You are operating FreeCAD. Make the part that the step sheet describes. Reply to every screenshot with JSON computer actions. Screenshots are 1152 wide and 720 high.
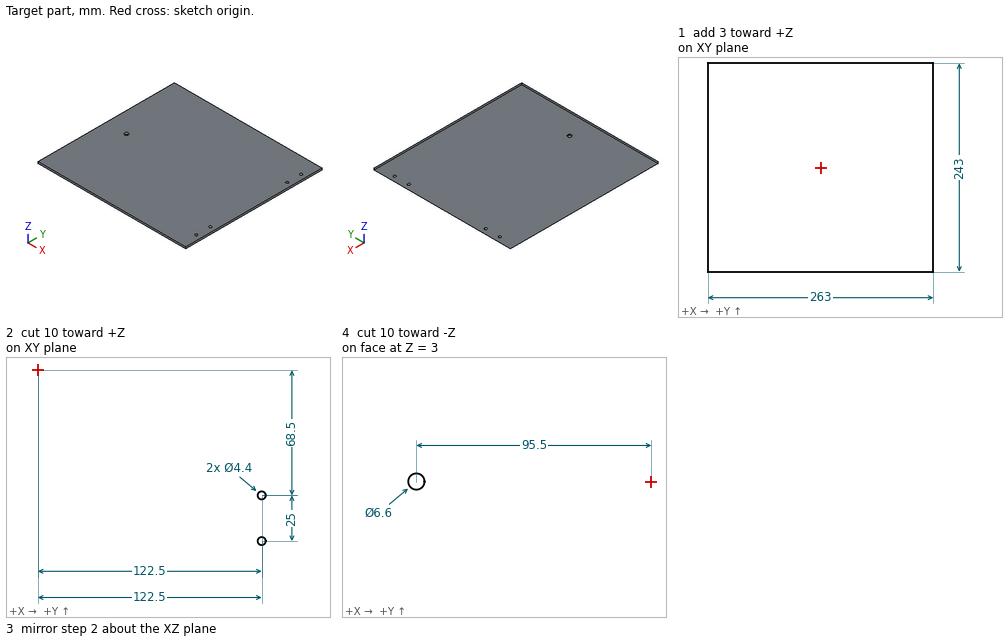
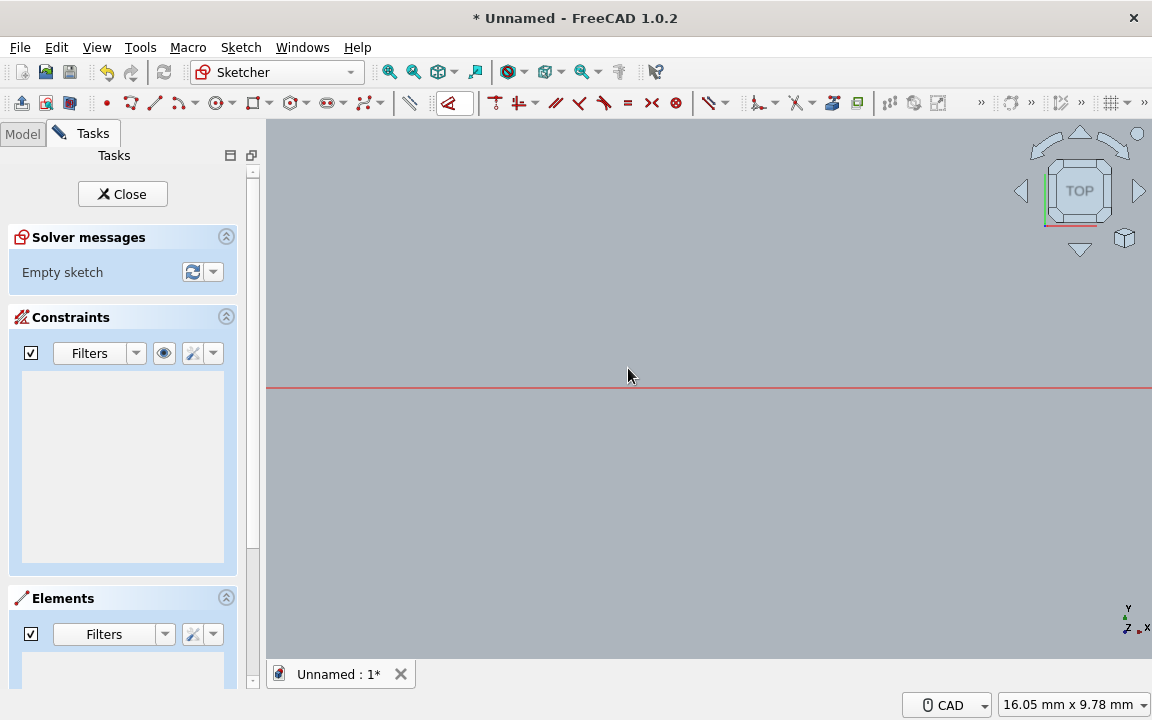
{"action": "key", "text": "g c"}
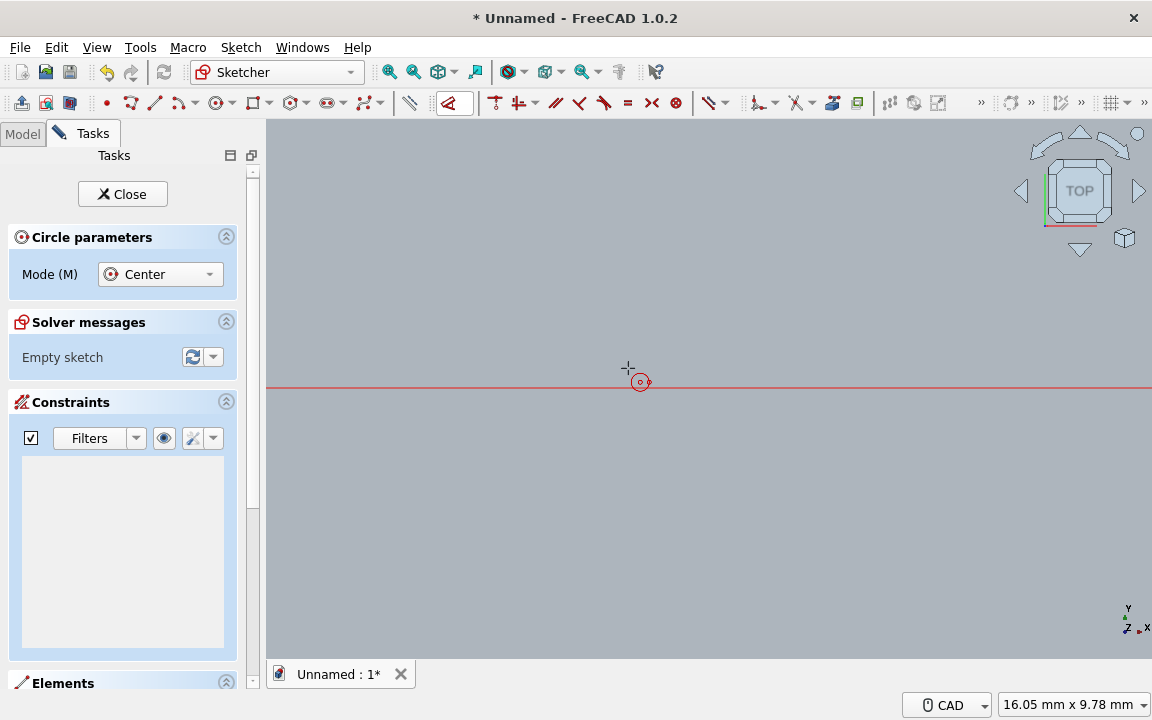
{"action": "left_click", "coordinate": [640, 388]}
{"action": "left_click", "coordinate": [769, 260]}
{"action": "key", "text": "Escape"}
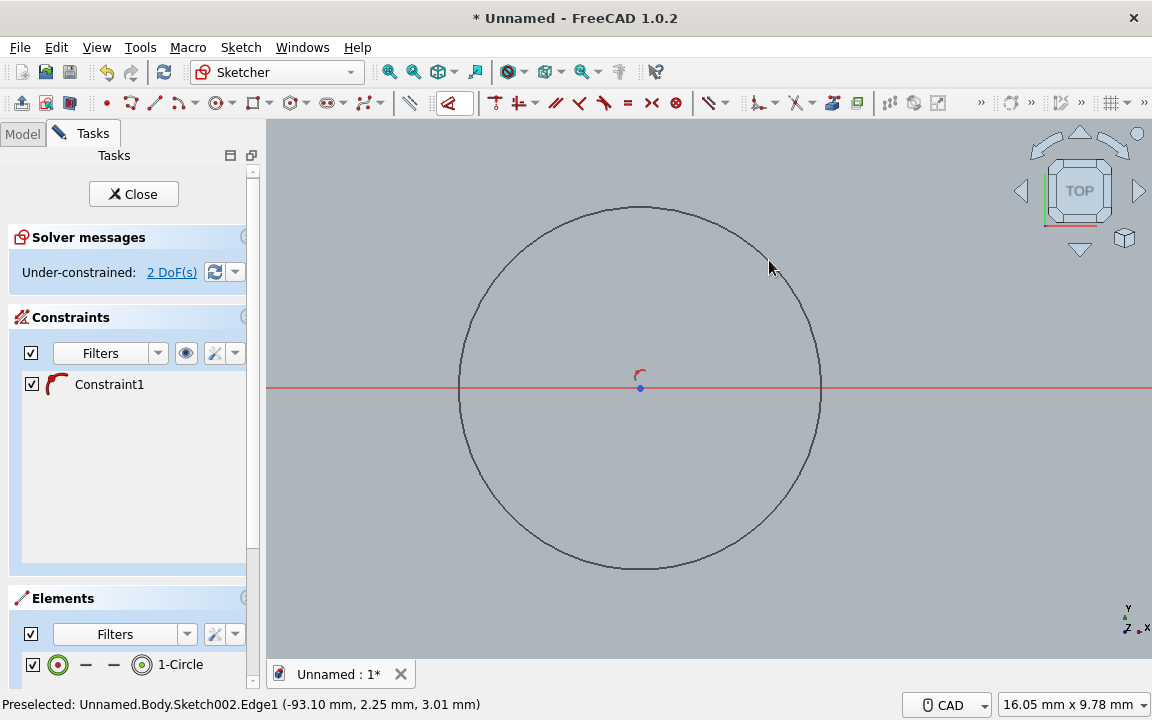
{"action": "left_click", "coordinate": [768, 260]}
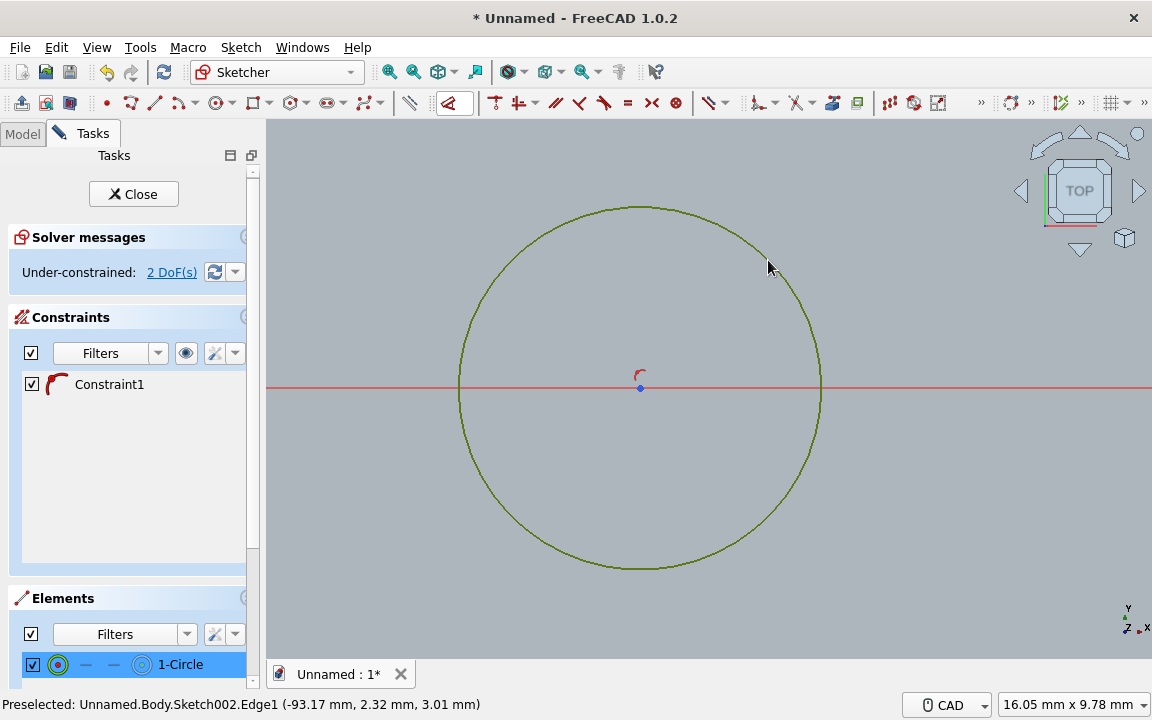
{"action": "key", "text": "k o"}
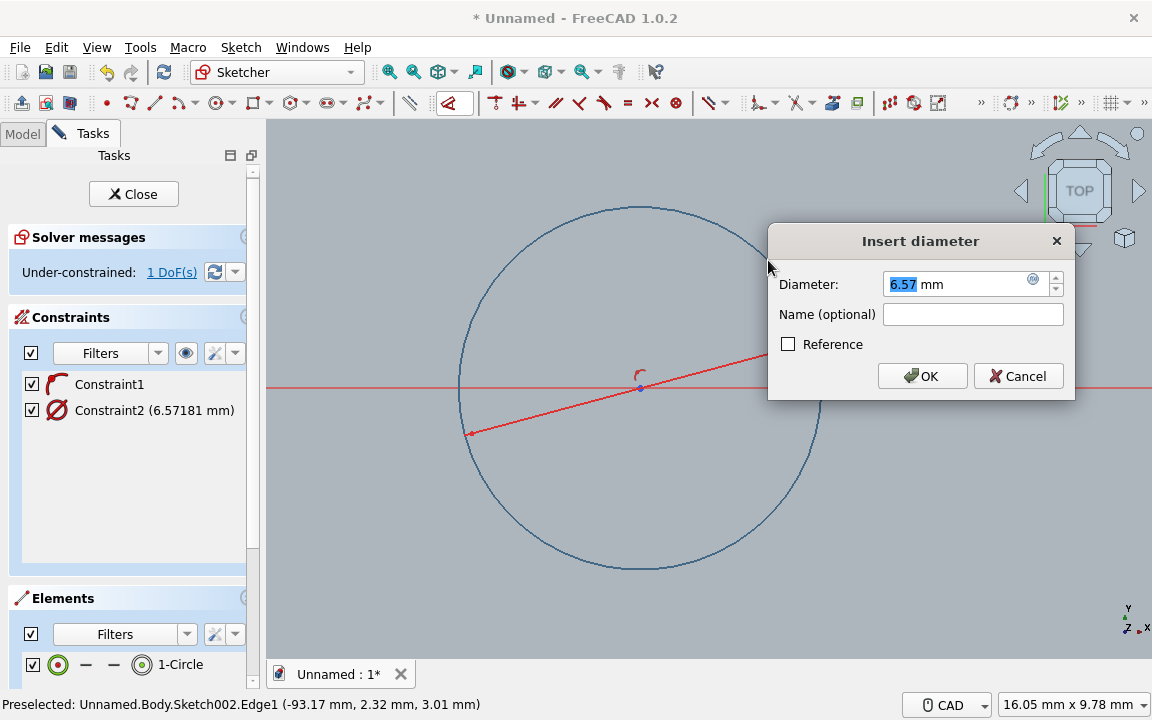
{"action": "type", "text": "6.6"}
{"action": "key", "text": "Return"}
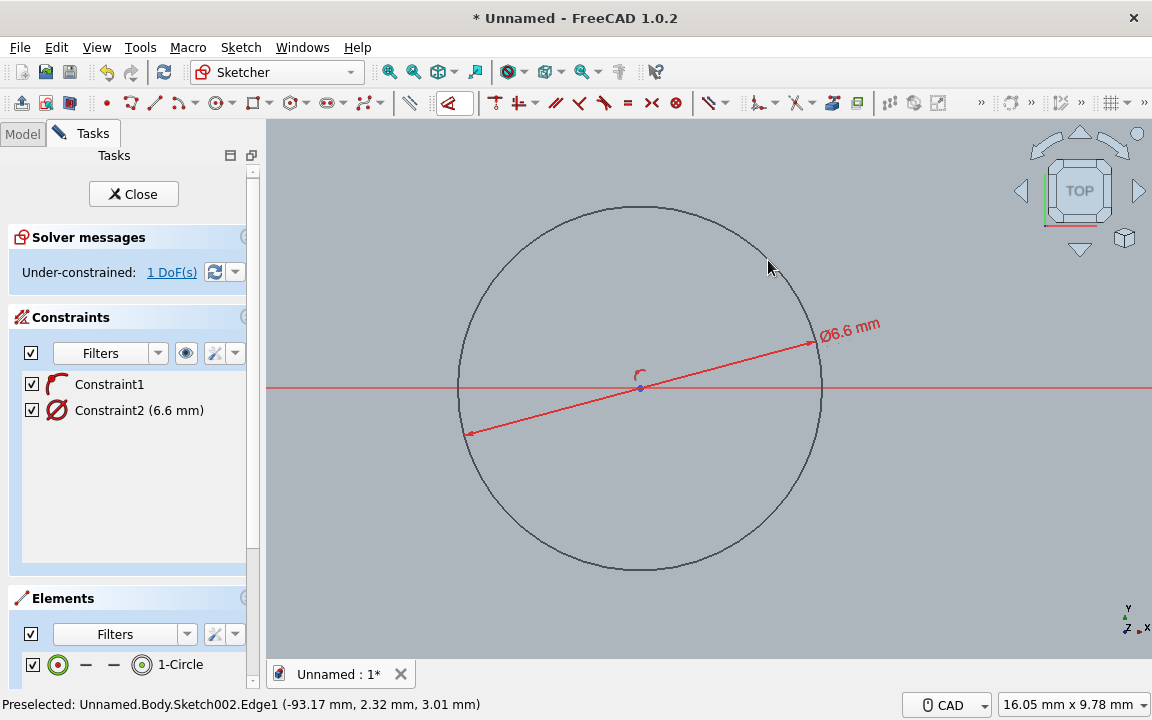
{"action": "left_click", "coordinate": [640, 388]}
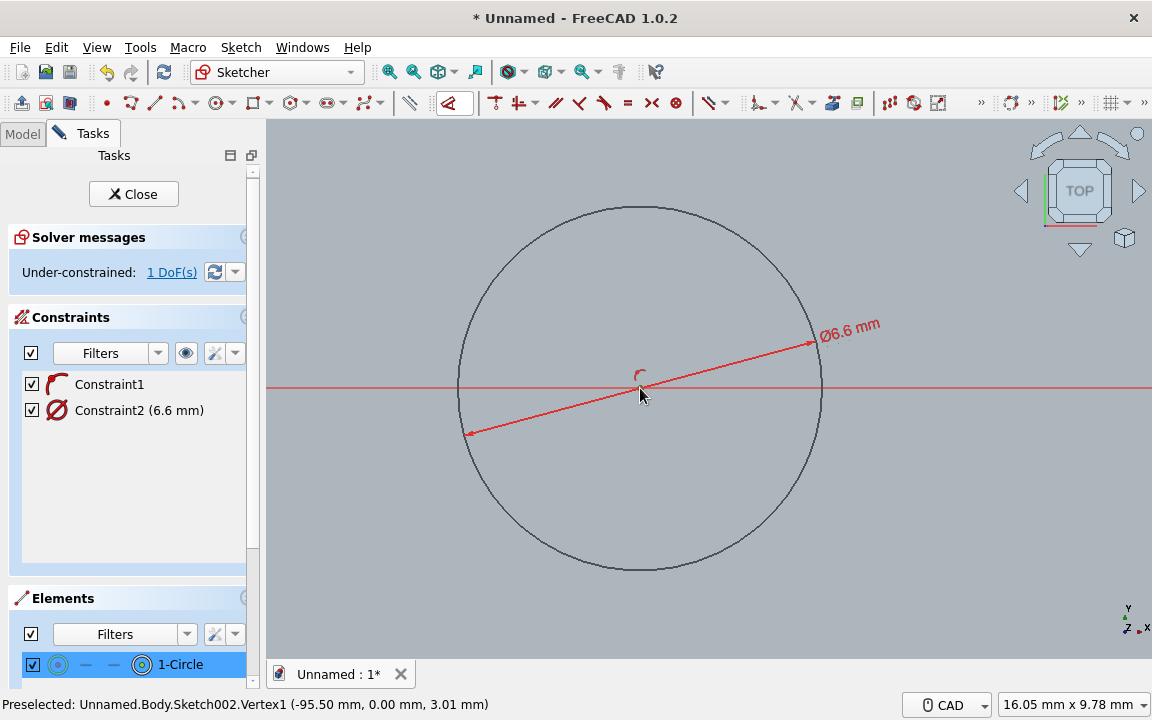
{"action": "key", "text": "l"}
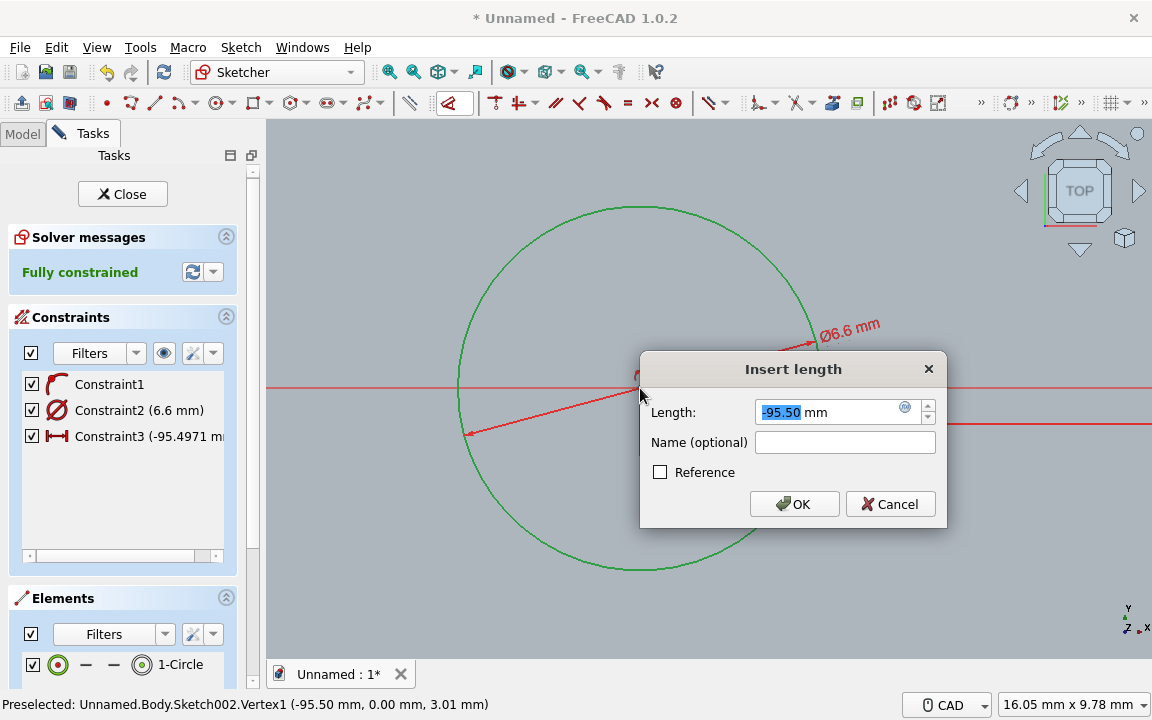
{"action": "type", "text": "-95.5"}
{"action": "key", "text": "Return"}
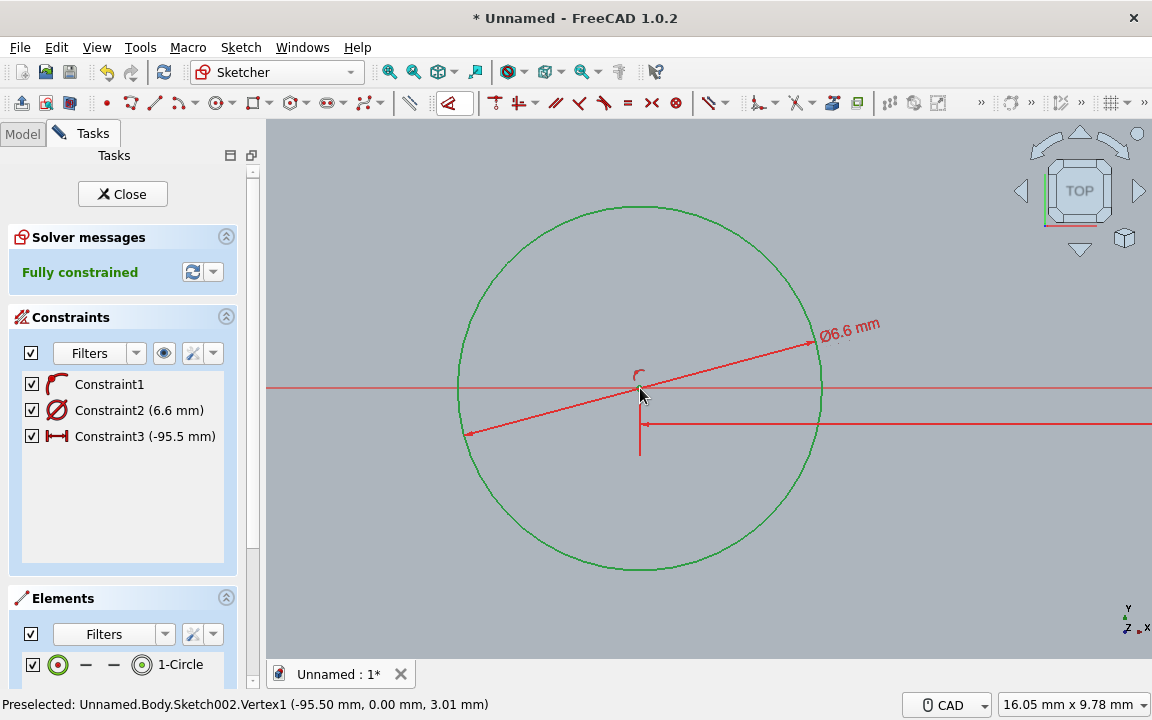
{"action": "left_click", "coordinate": [123, 194]}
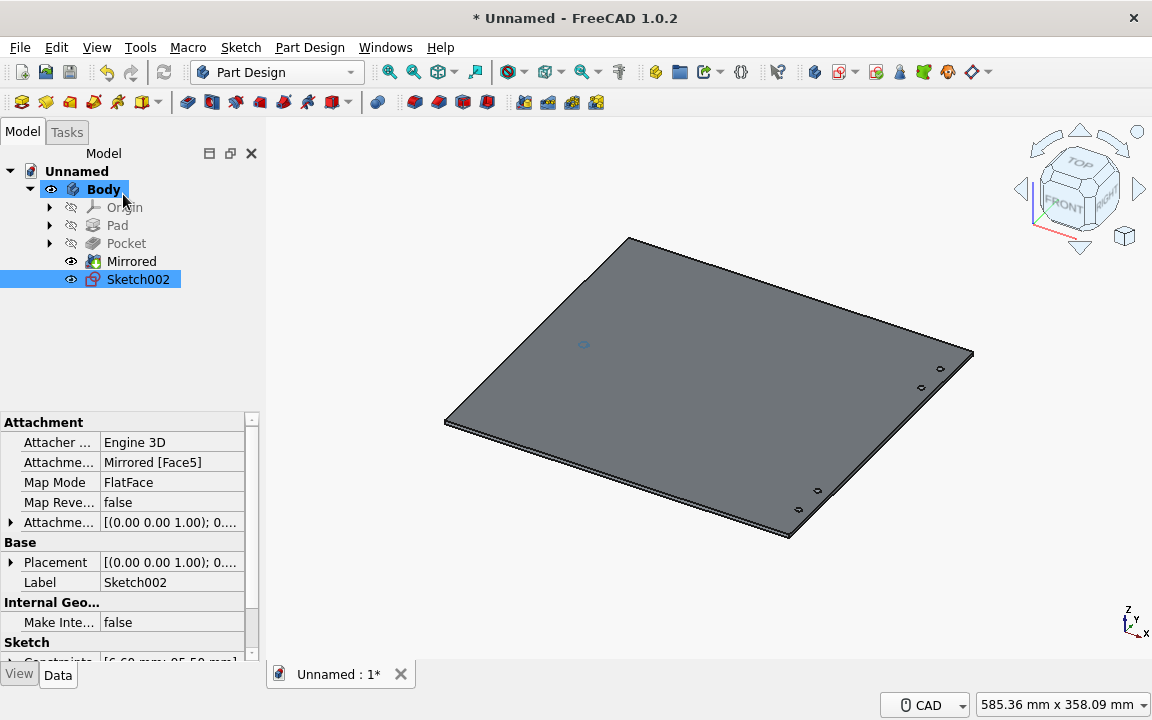
{"action": "left_click", "coordinate": [188, 102]}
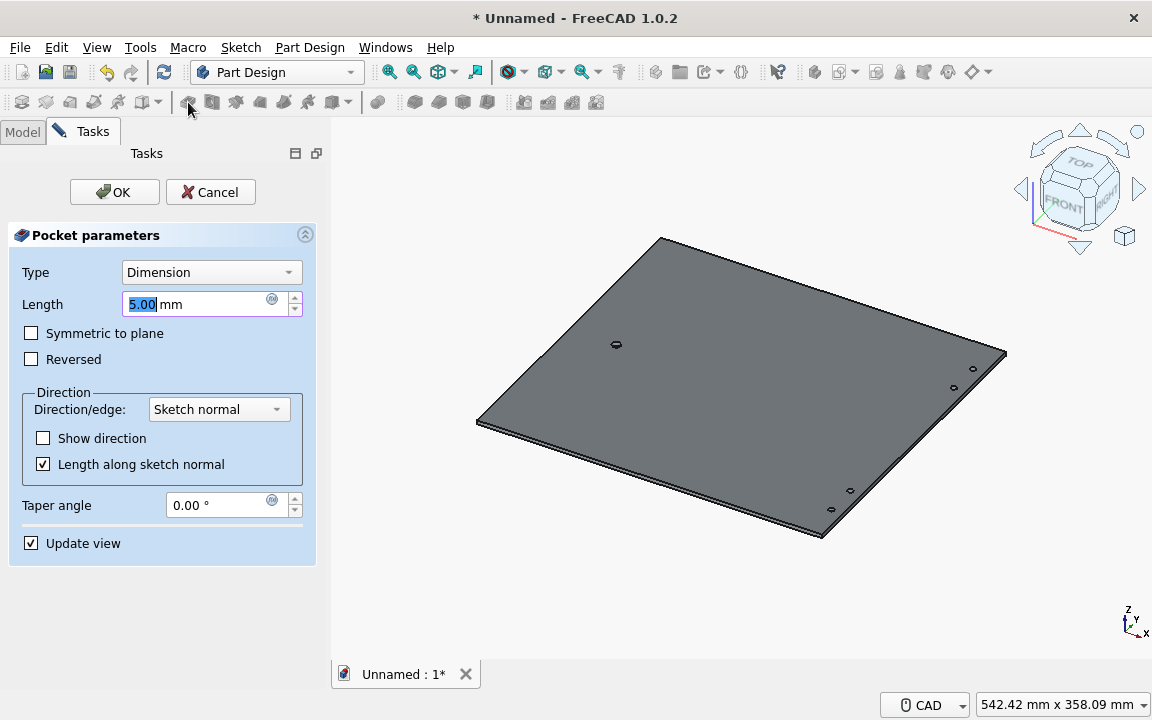
{"action": "type", "text": "10"}
{"action": "key", "text": "Tab"}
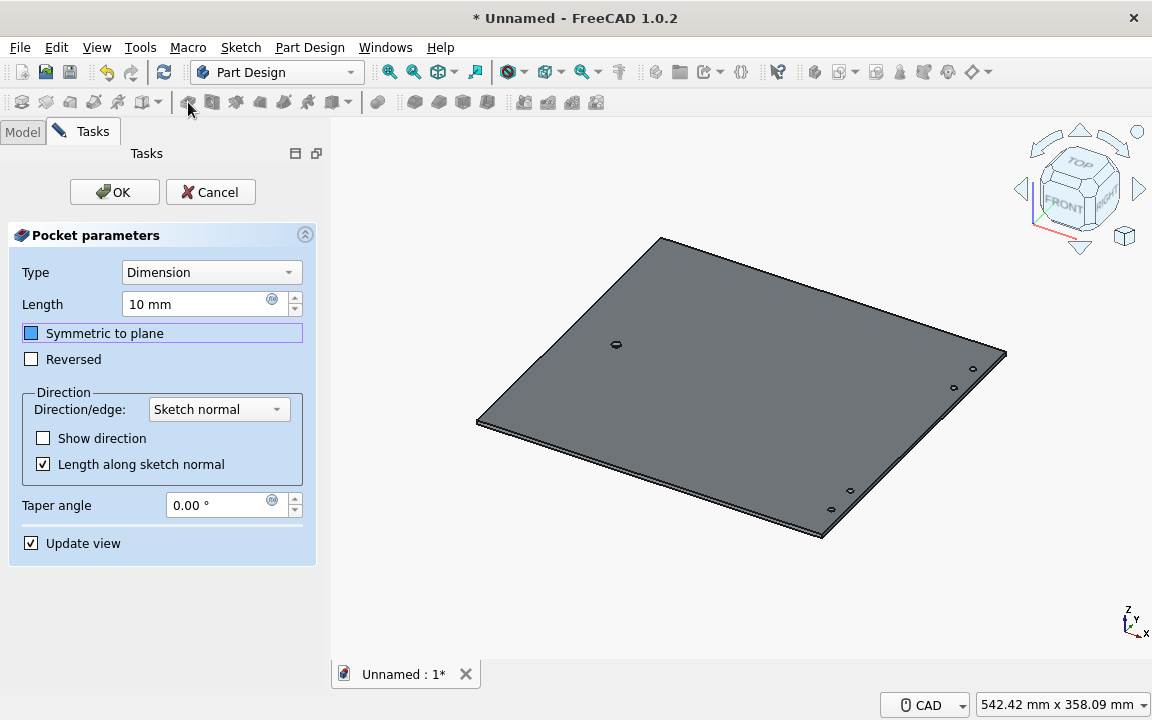
{"action": "left_click", "coordinate": [115, 192]}